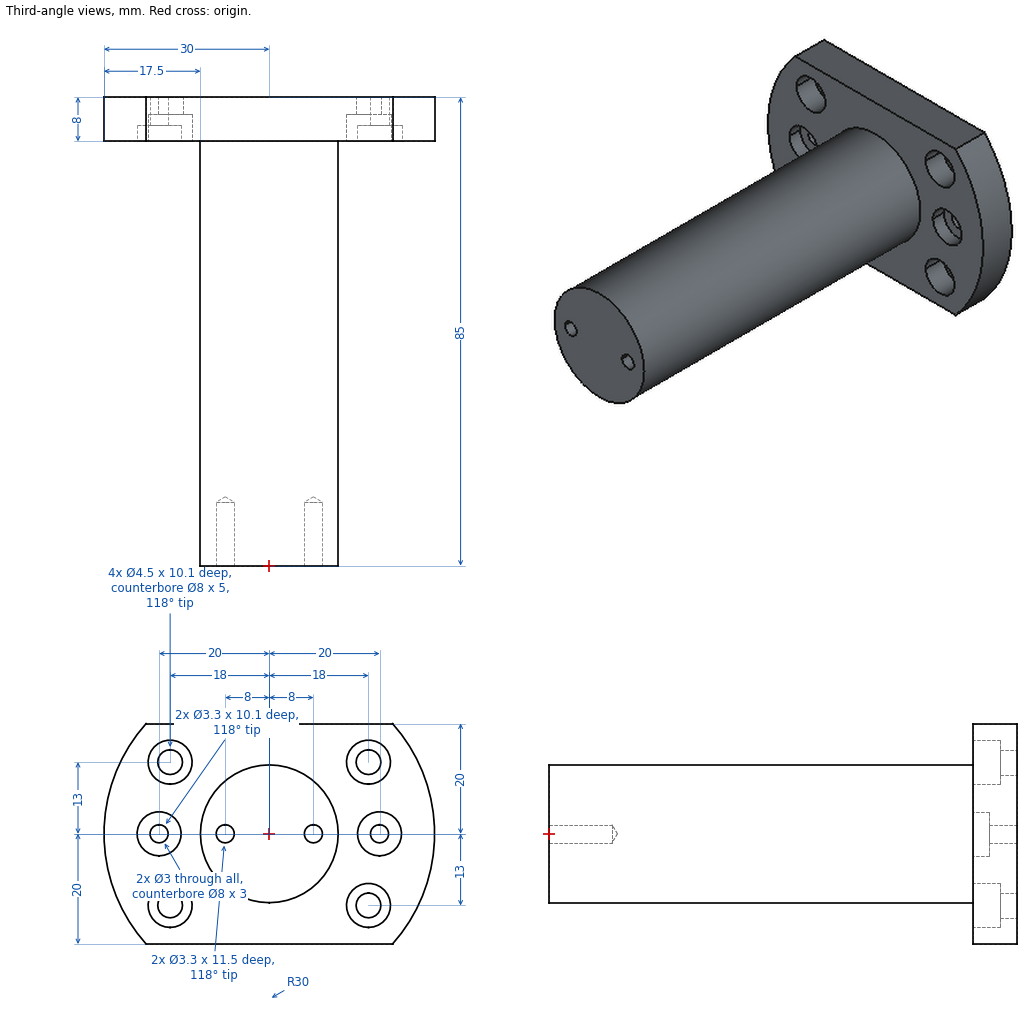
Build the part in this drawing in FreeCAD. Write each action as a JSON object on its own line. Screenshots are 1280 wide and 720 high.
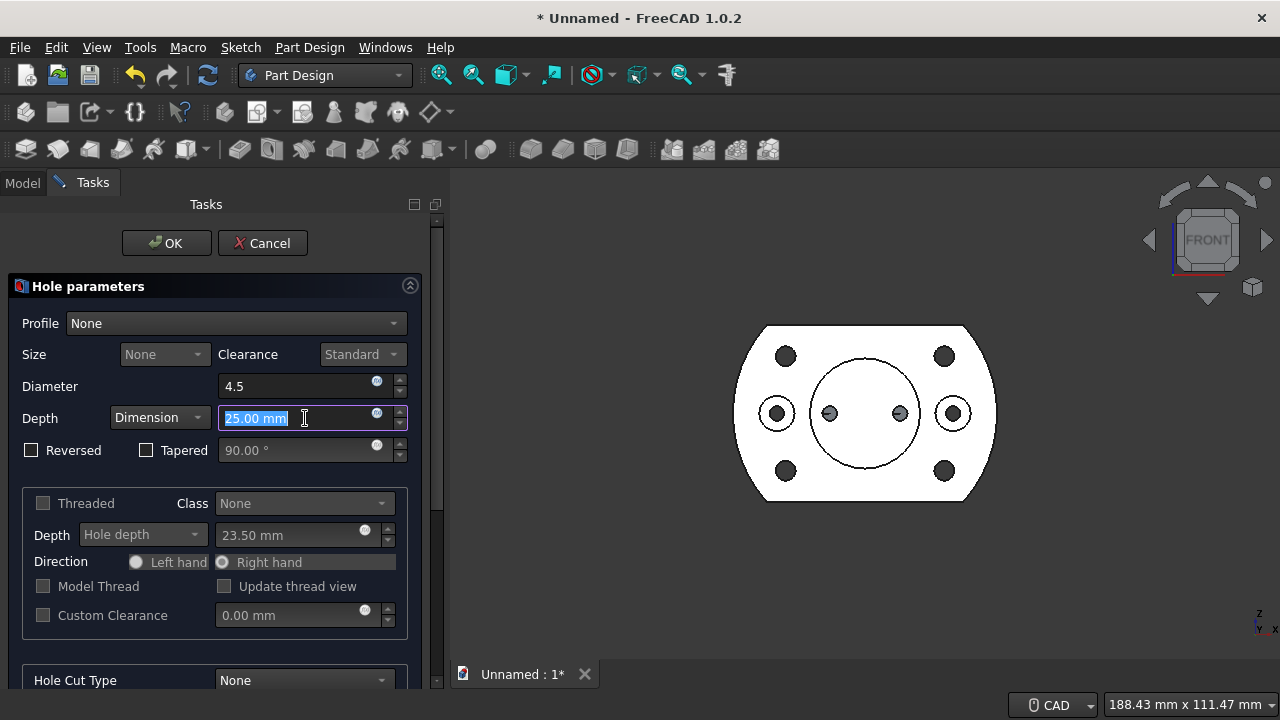
{"action": "type", "text": "10.1"}
{"action": "key", "text": "Tab"}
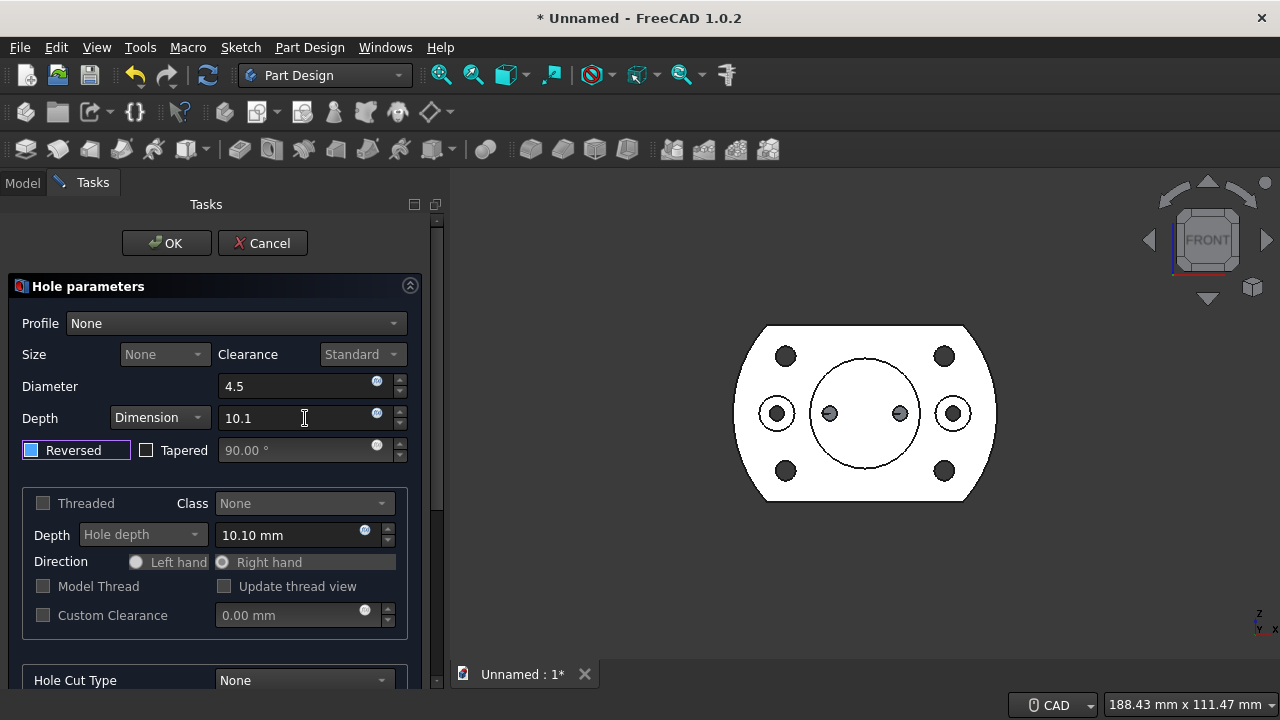
{"action": "scroll", "coordinate": [437, 451], "scroll_direction": "down", "scroll_amount": 2}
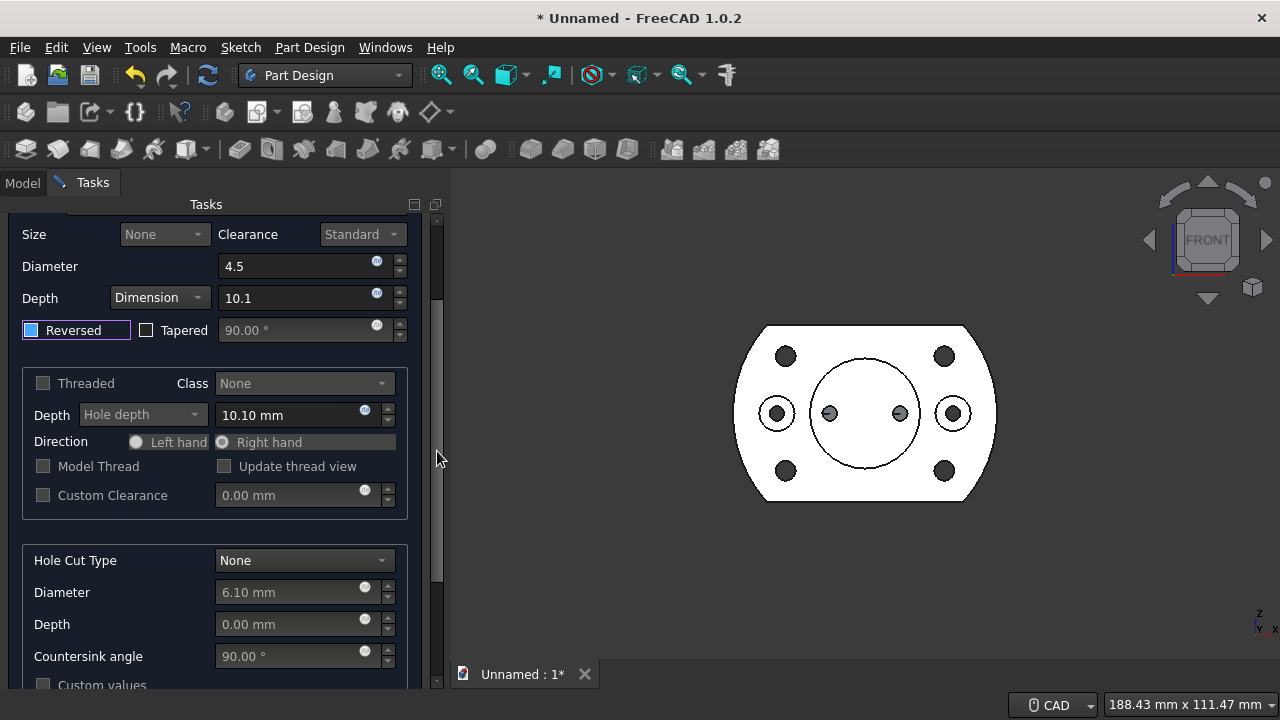
{"action": "left_click", "coordinate": [306, 560]}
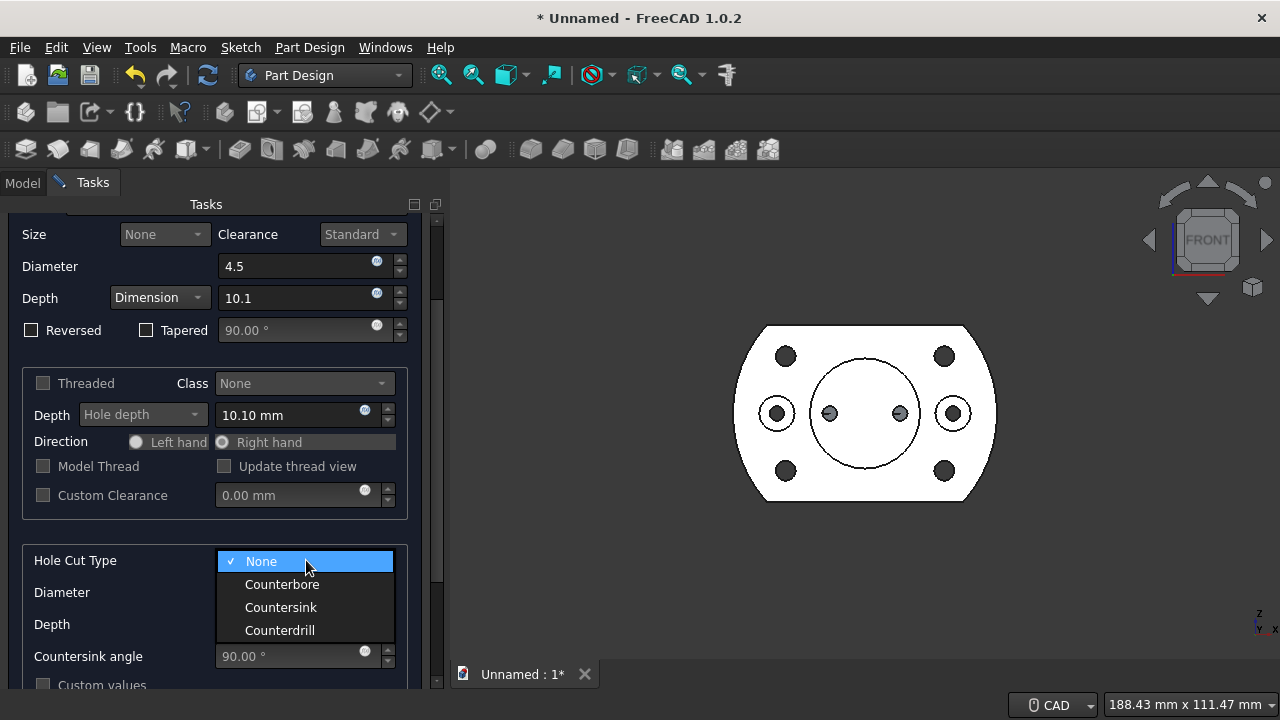
{"action": "left_click", "coordinate": [304, 584]}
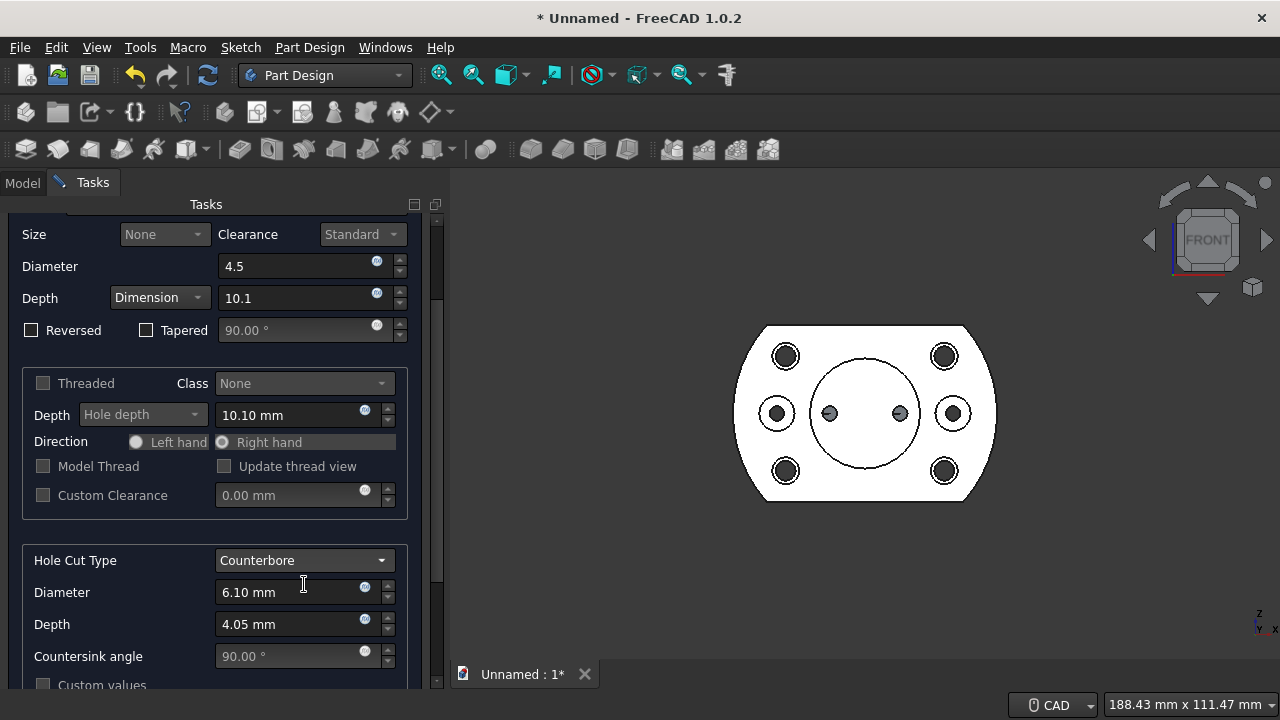
{"action": "triple_click", "coordinate": [298, 592]}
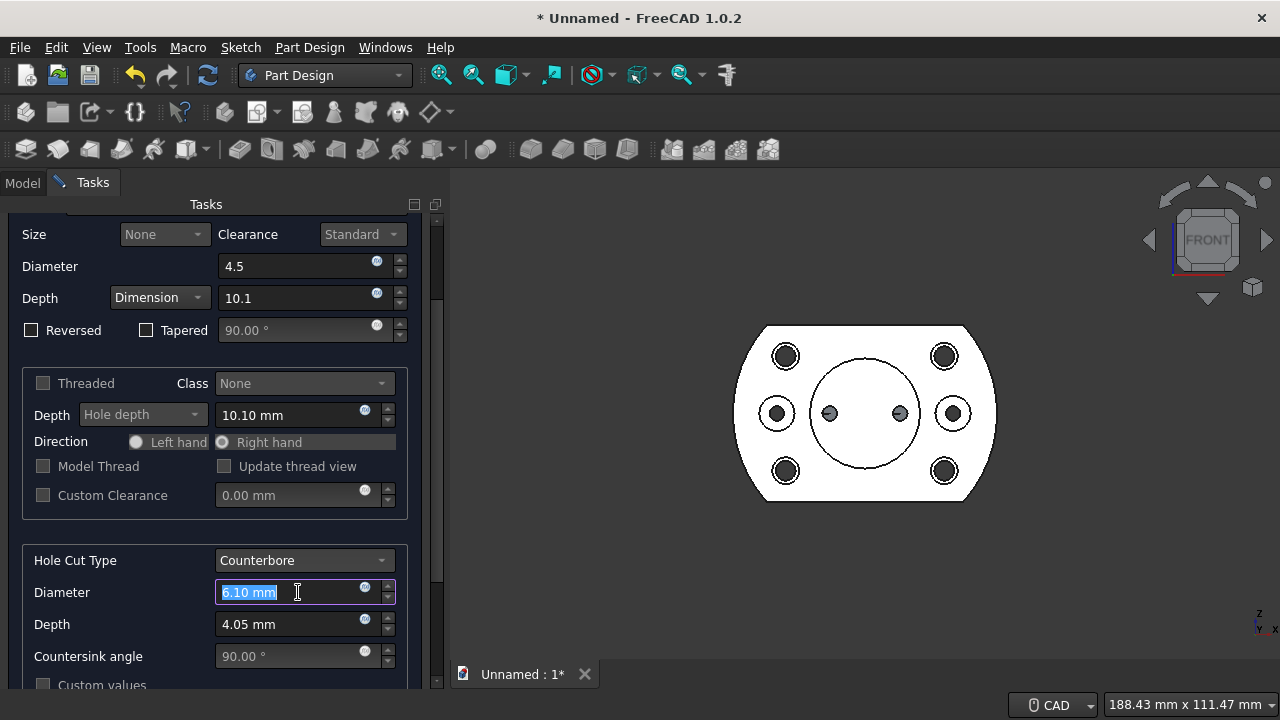
{"action": "type", "text": "8"}
{"action": "key", "text": "Tab"}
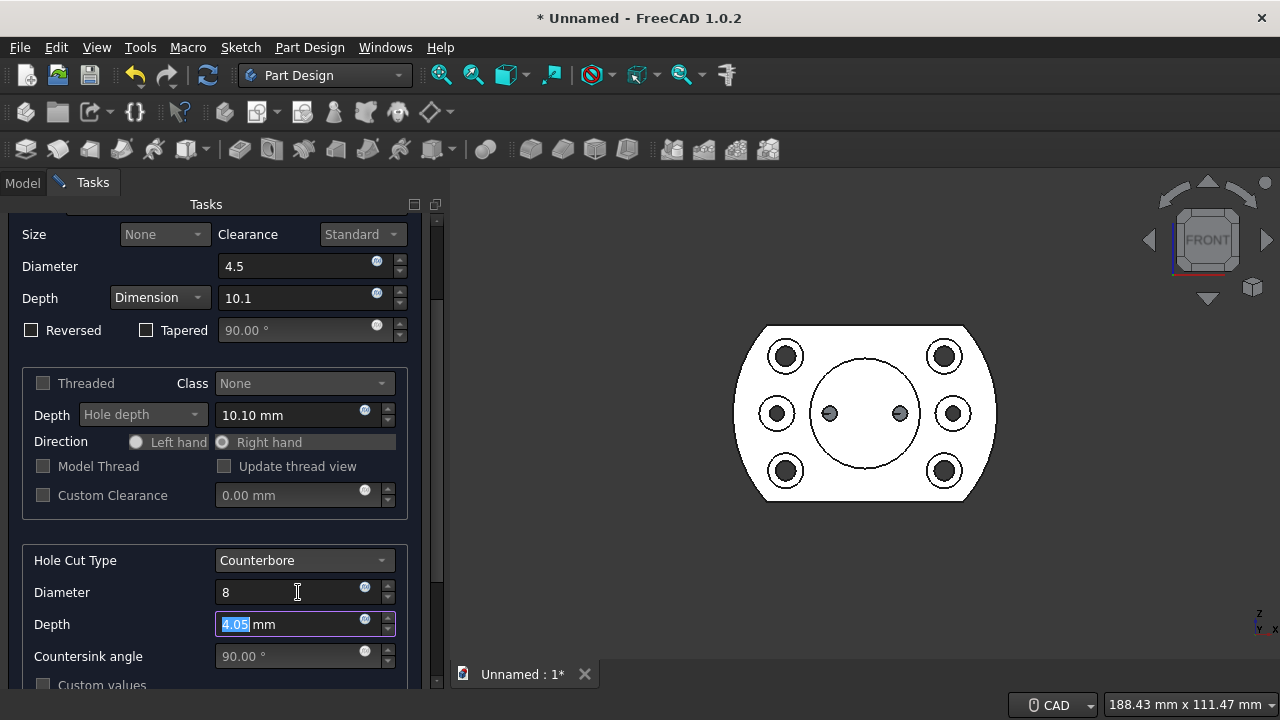
{"action": "type", "text": "5"}
{"action": "key", "text": "Tab"}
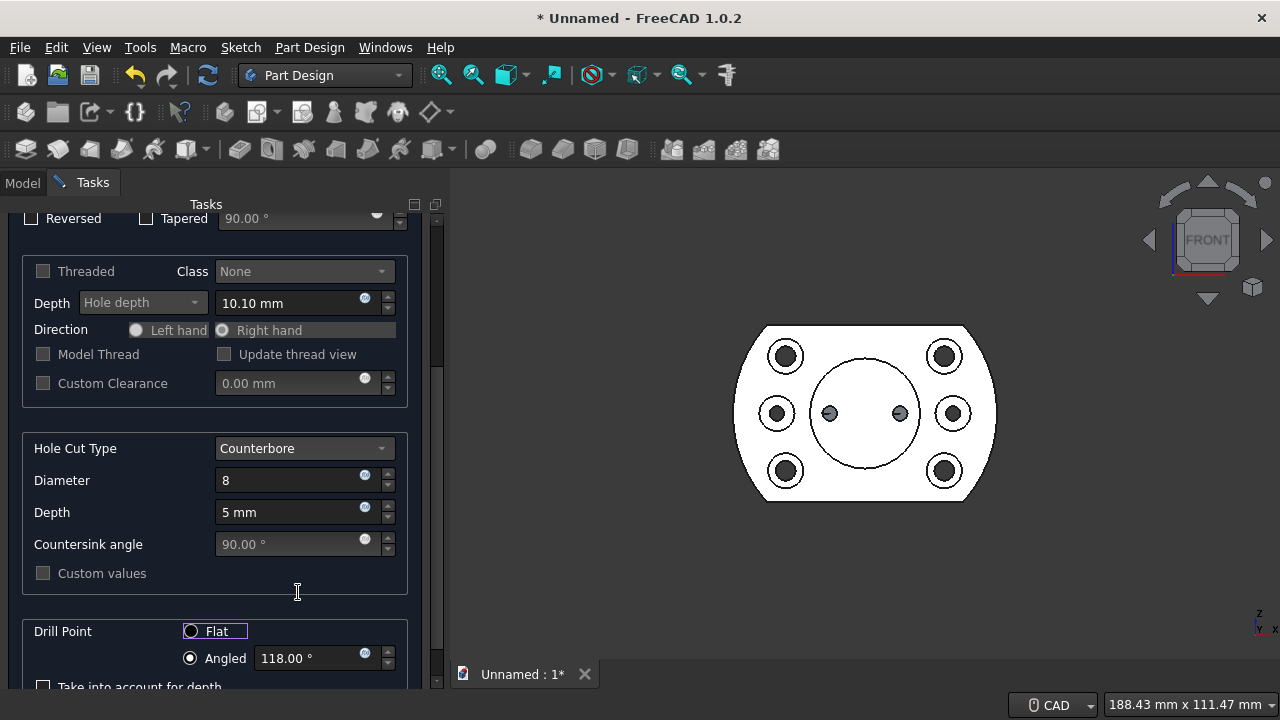
{"action": "scroll", "coordinate": [437, 451], "scroll_direction": "up", "scroll_amount": 5}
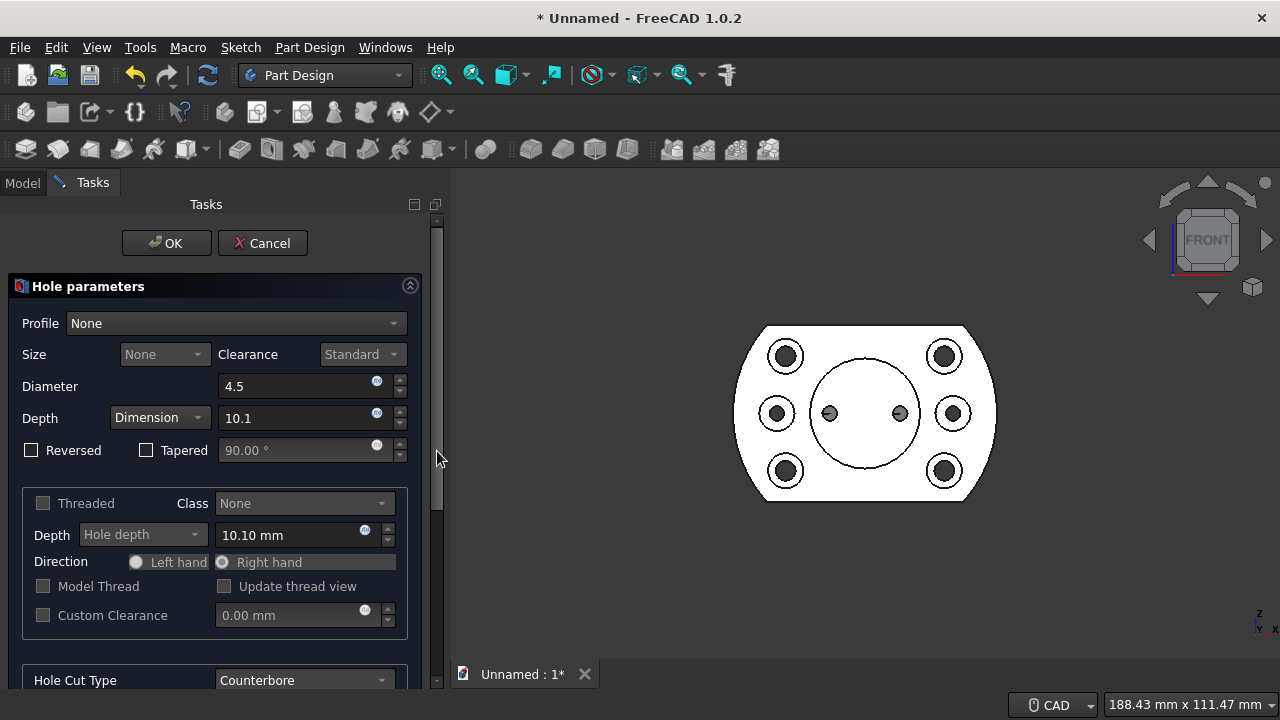
{"action": "left_click", "coordinate": [167, 243]}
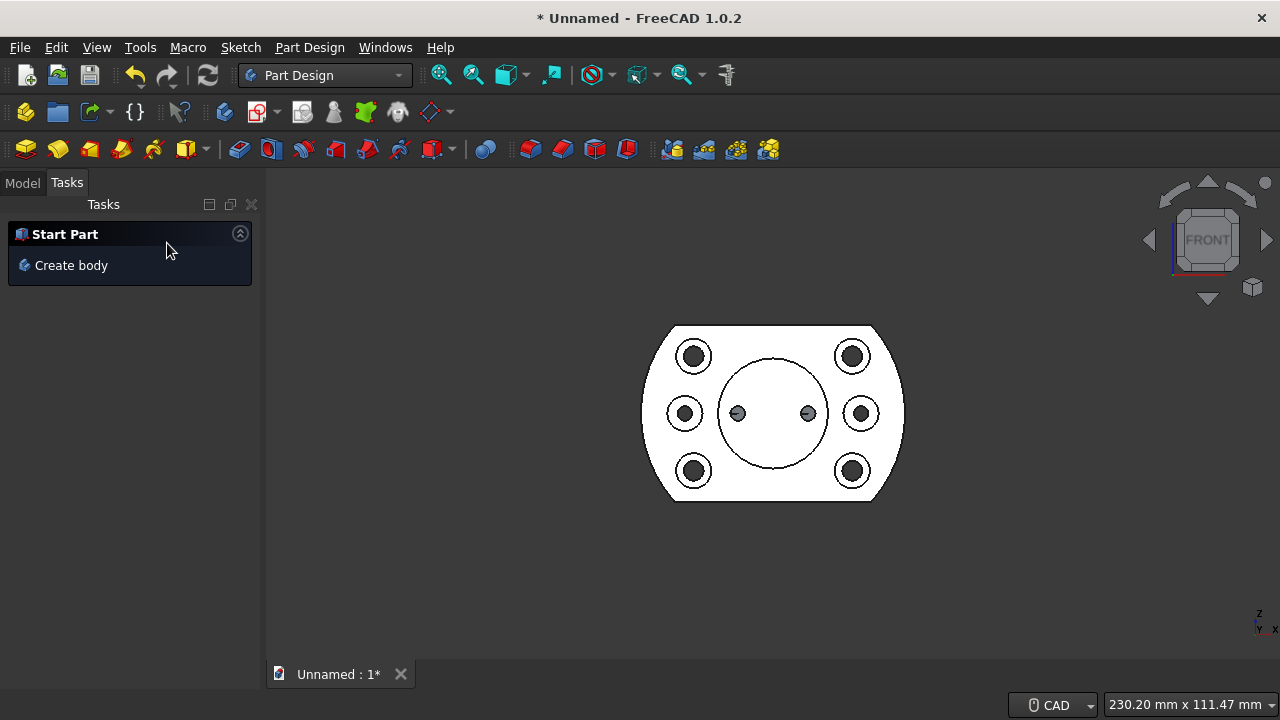
{"action": "key", "text": "0"}